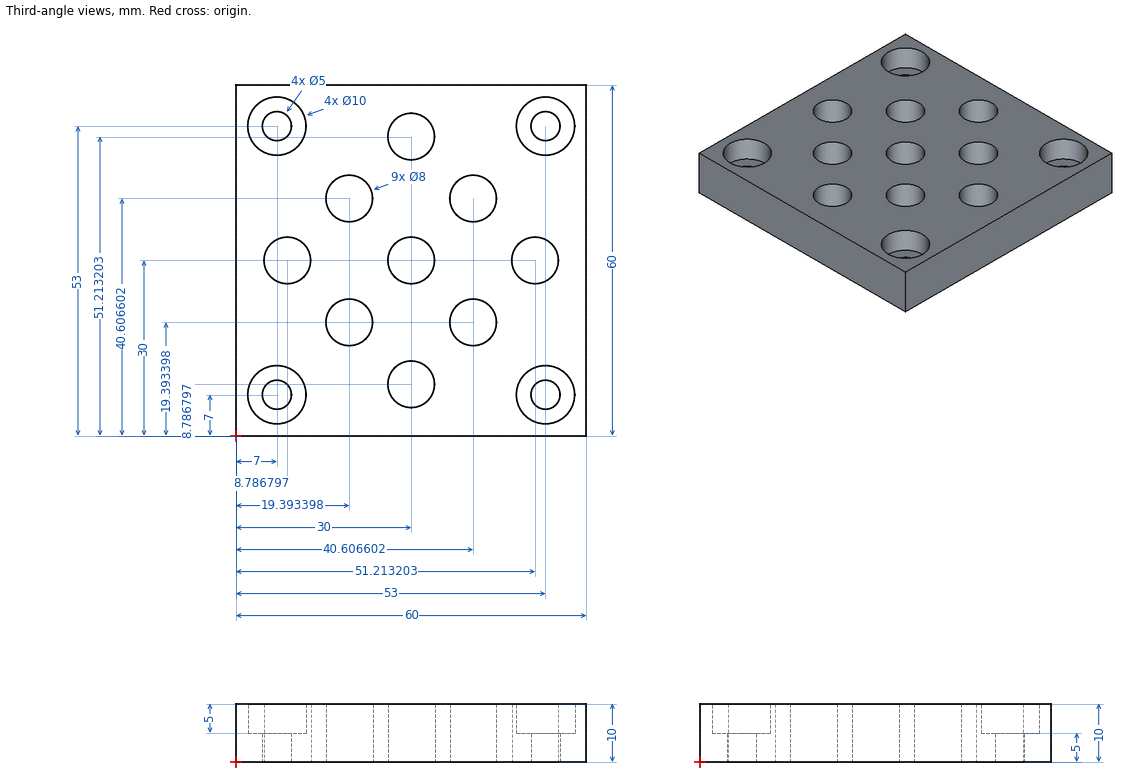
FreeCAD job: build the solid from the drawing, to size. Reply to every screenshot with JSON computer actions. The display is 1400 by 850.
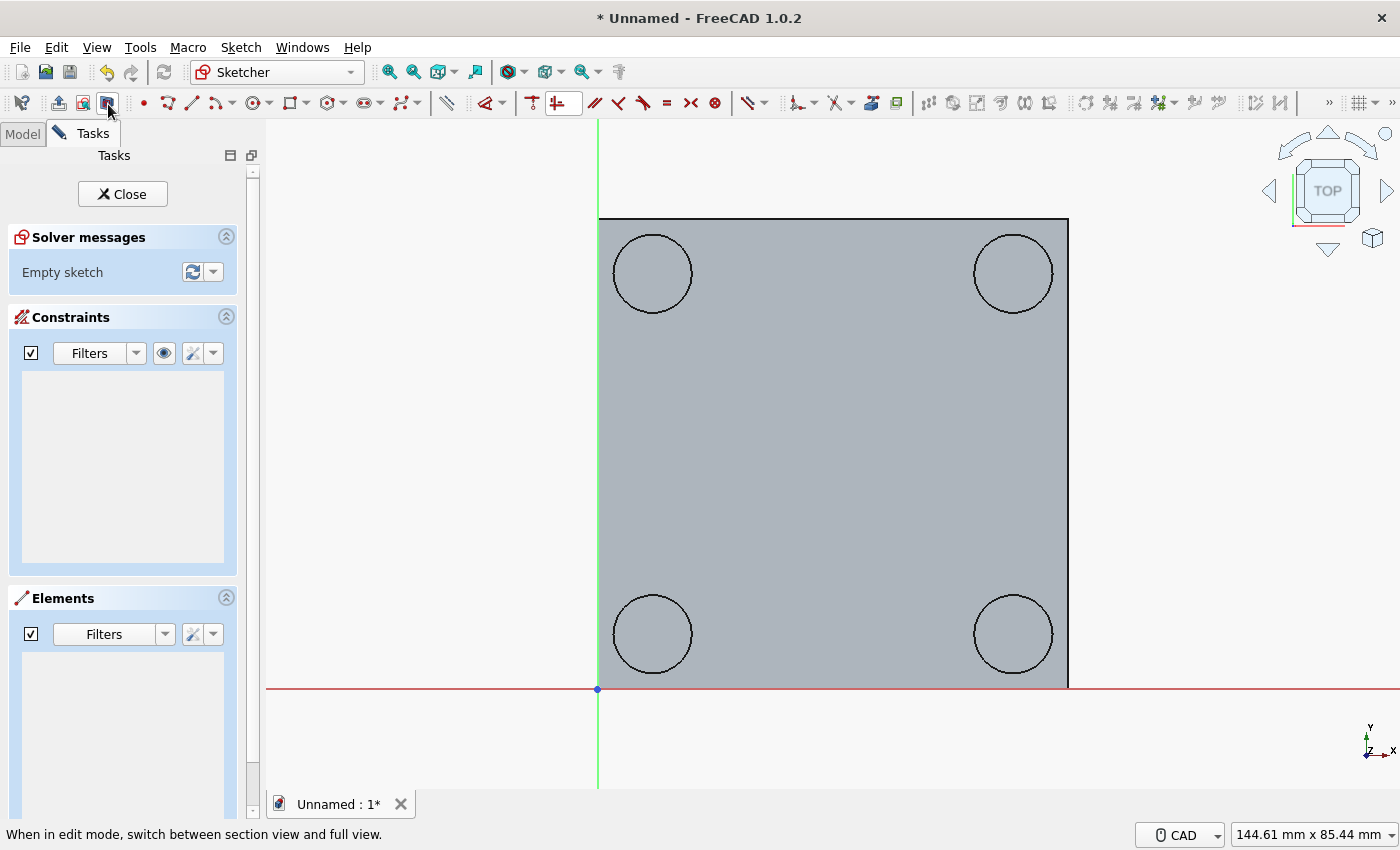
{"action": "key", "text": "g c"}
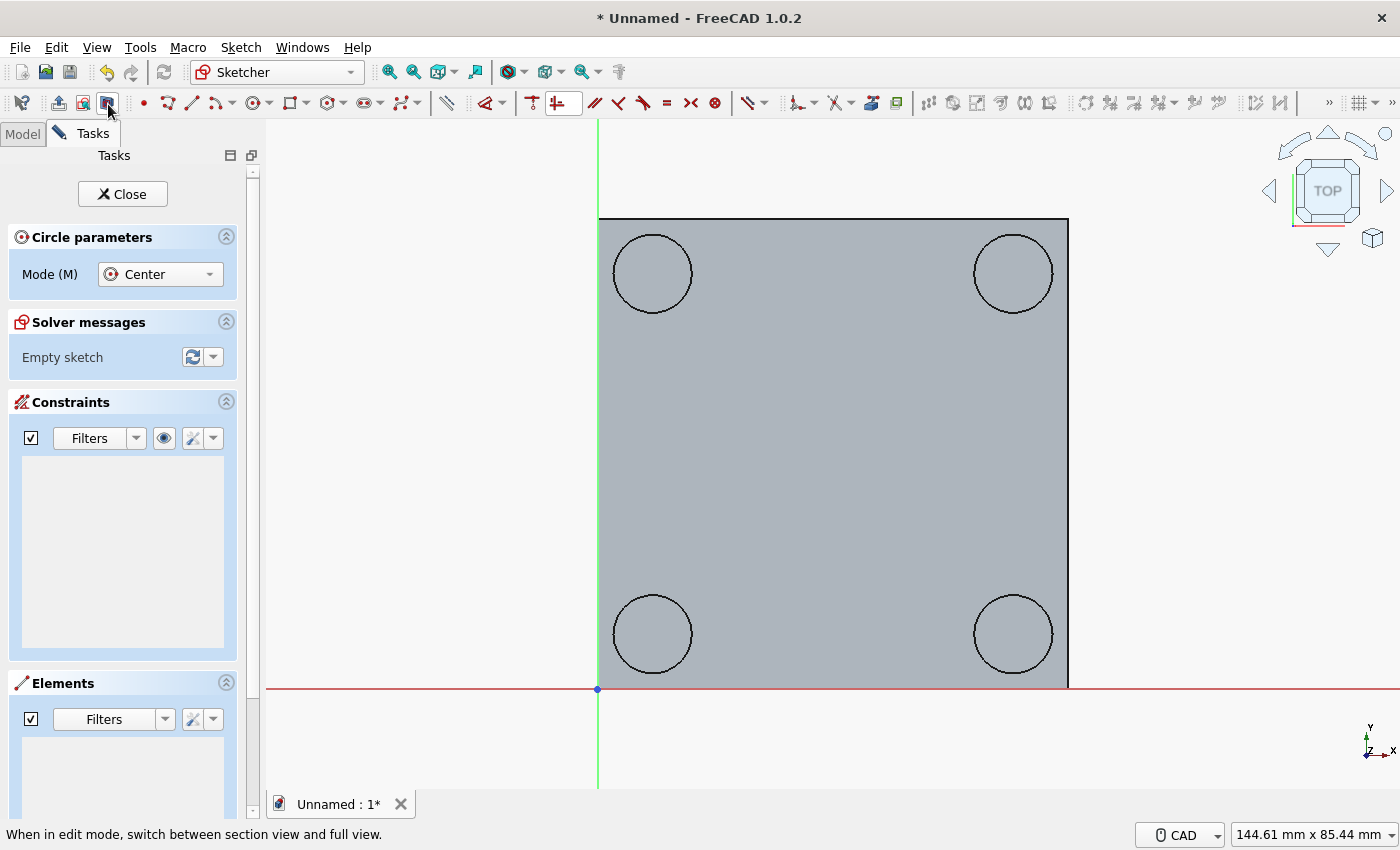
{"action": "left_click", "coordinate": [653, 274]}
{"action": "left_click", "coordinate": [667, 260]}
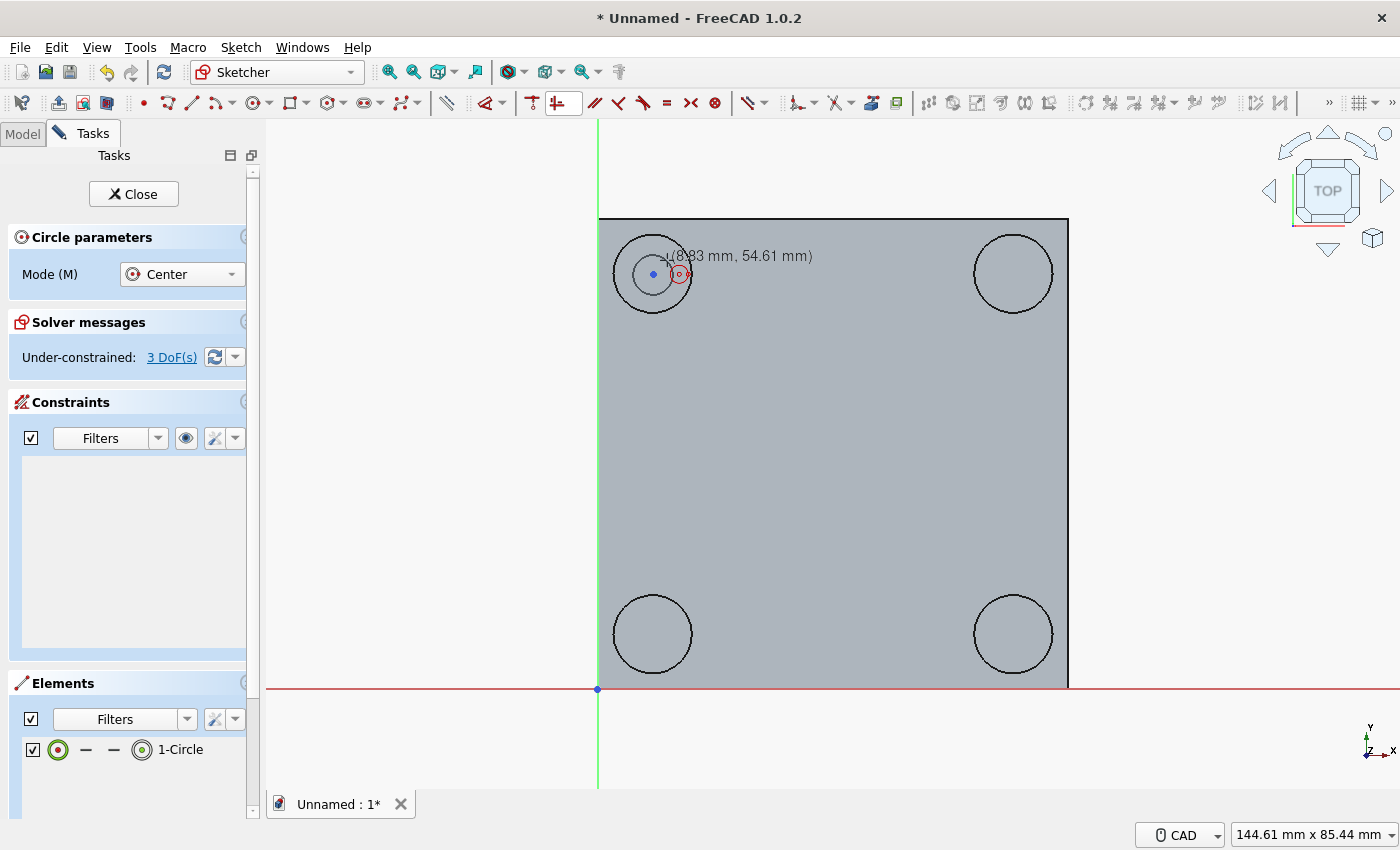
{"action": "left_click", "coordinate": [1013, 274]}
{"action": "left_click", "coordinate": [1027, 260]}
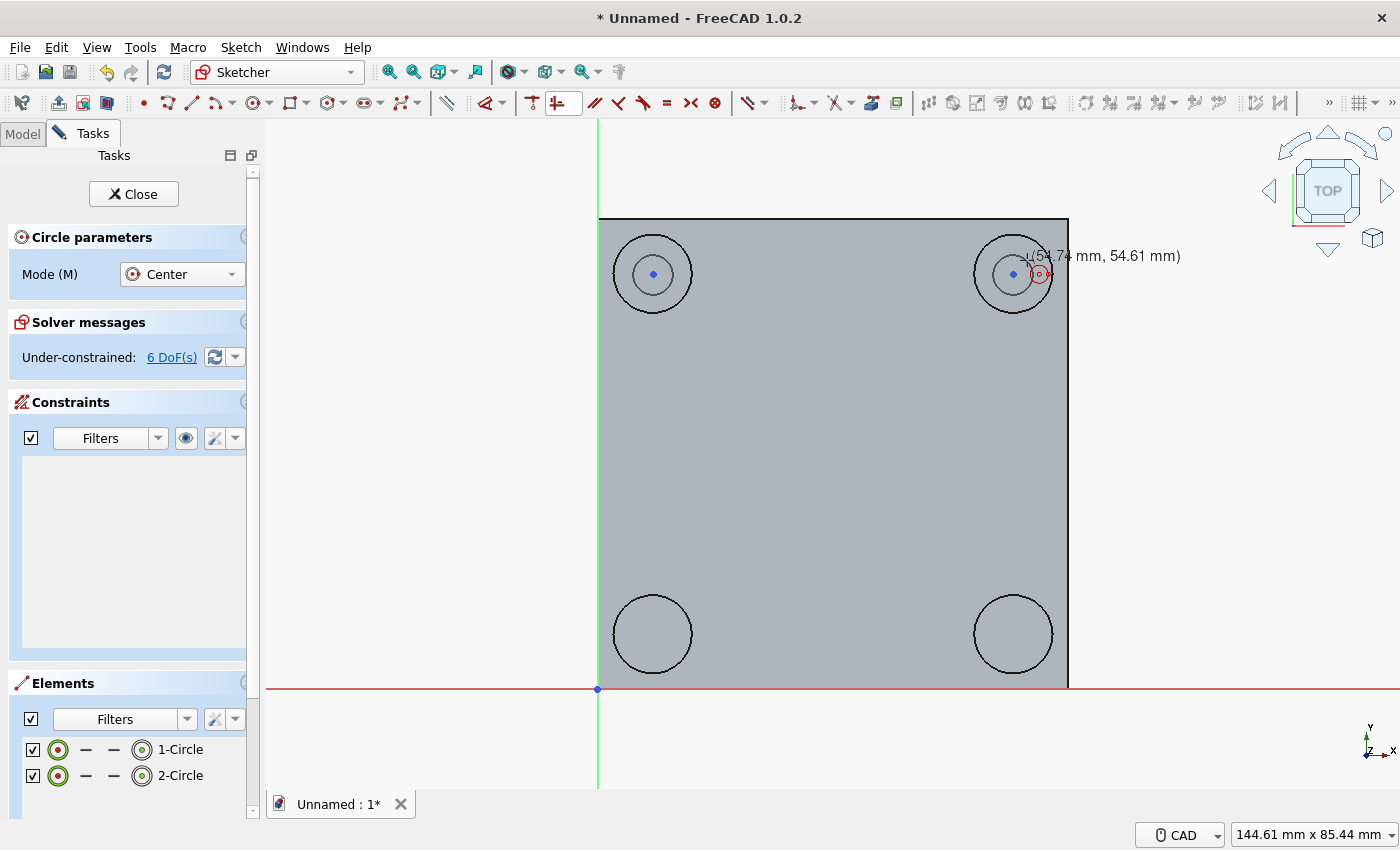
{"action": "left_click", "coordinate": [653, 634]}
{"action": "left_click", "coordinate": [667, 620]}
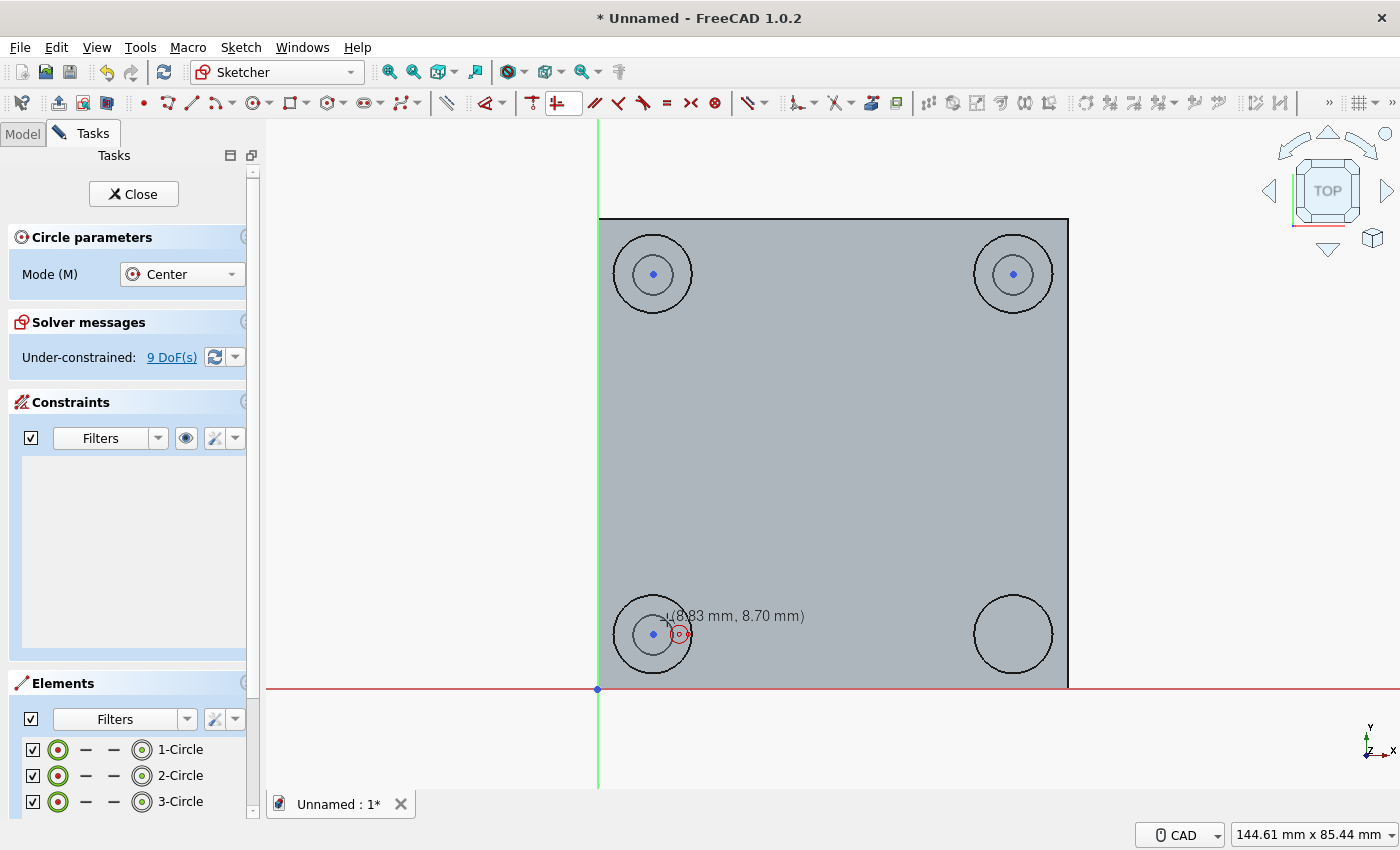
{"action": "left_click", "coordinate": [1013, 634]}
{"action": "left_click", "coordinate": [1027, 620]}
{"action": "key", "text": "Escape"}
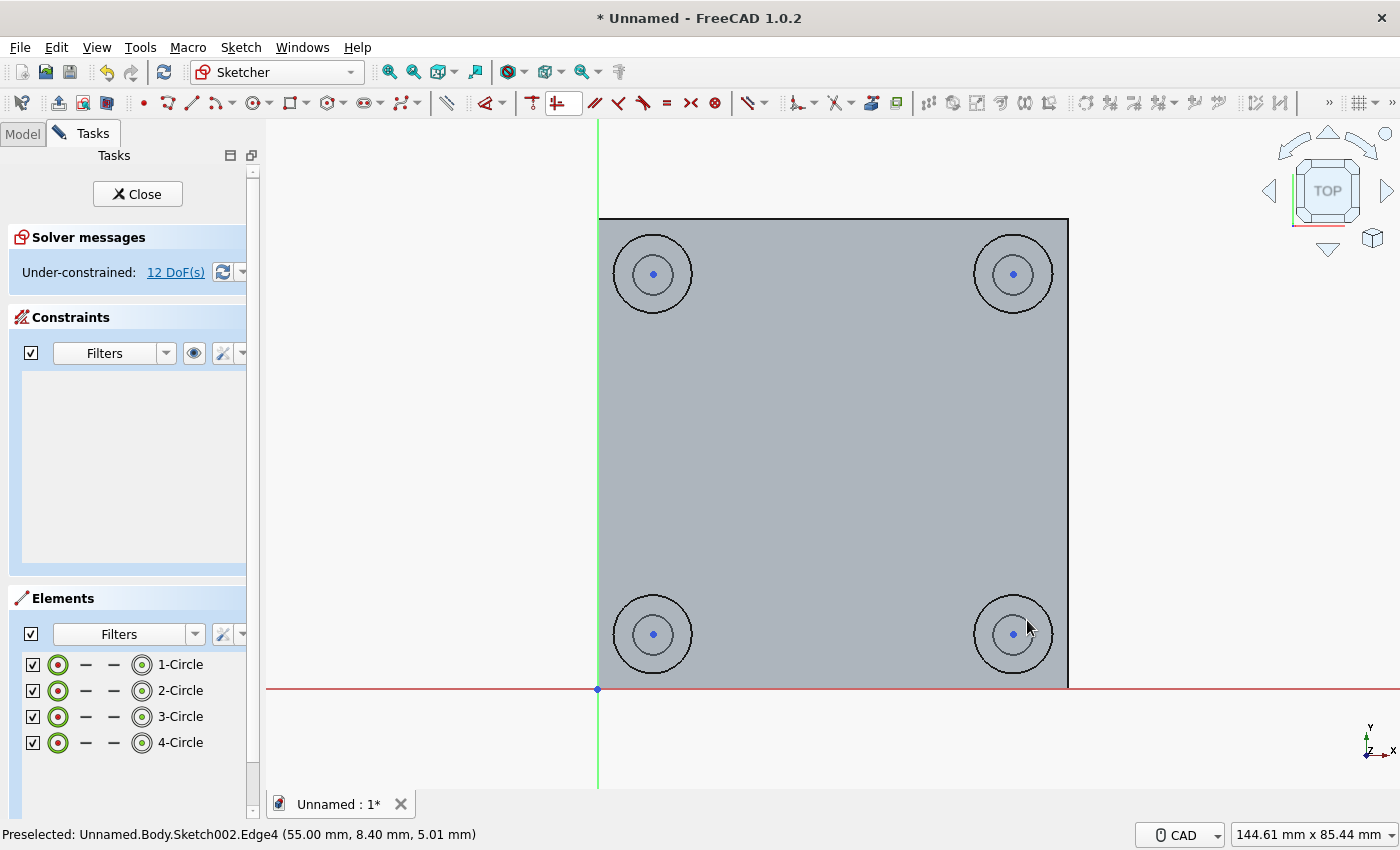
{"action": "left_click", "coordinate": [667, 261]}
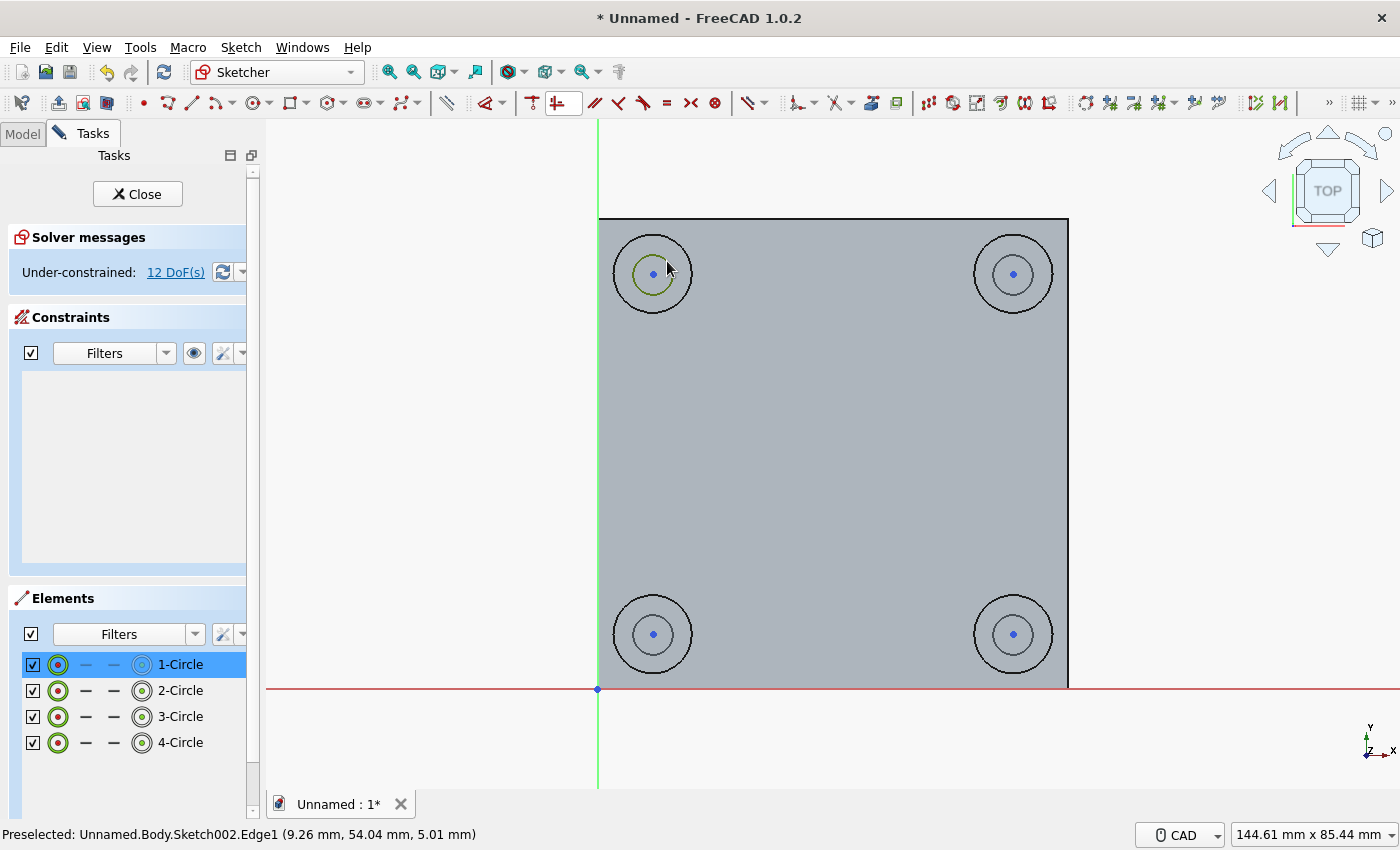
{"action": "left_click", "coordinate": [1027, 261]}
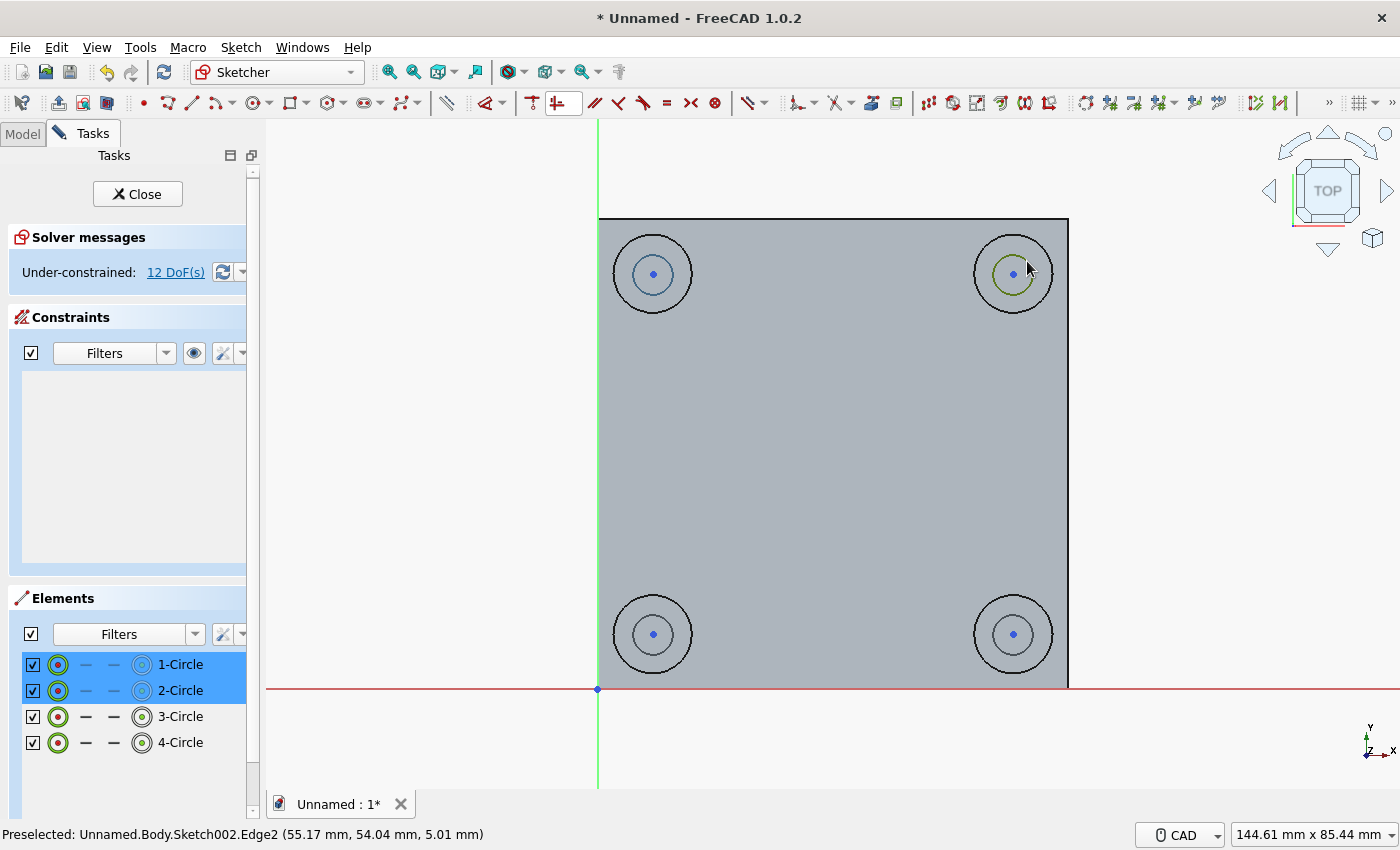
{"action": "left_click", "coordinate": [667, 621]}